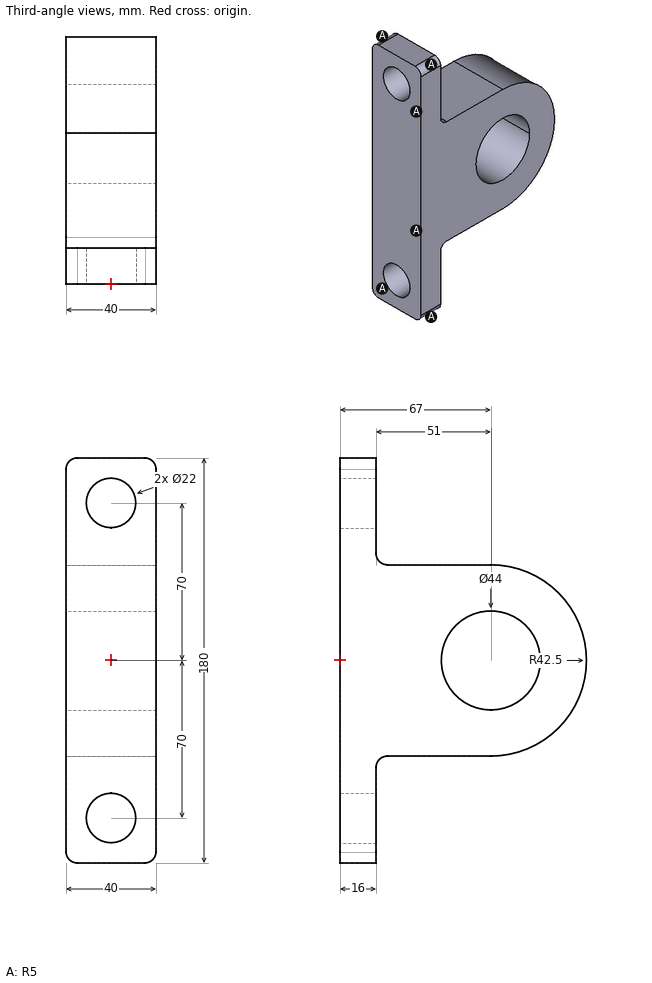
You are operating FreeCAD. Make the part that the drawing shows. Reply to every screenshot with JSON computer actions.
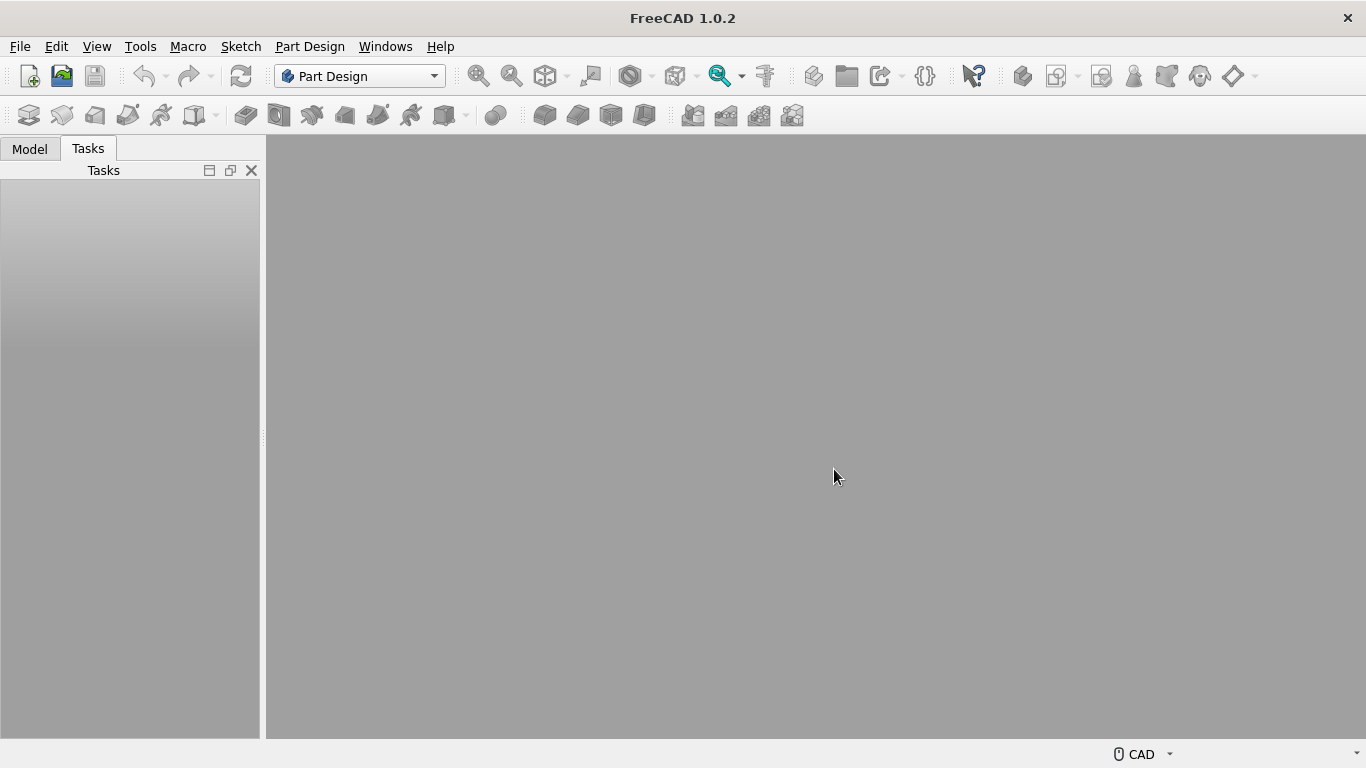
{"action": "left_click", "coordinate": [29, 76]}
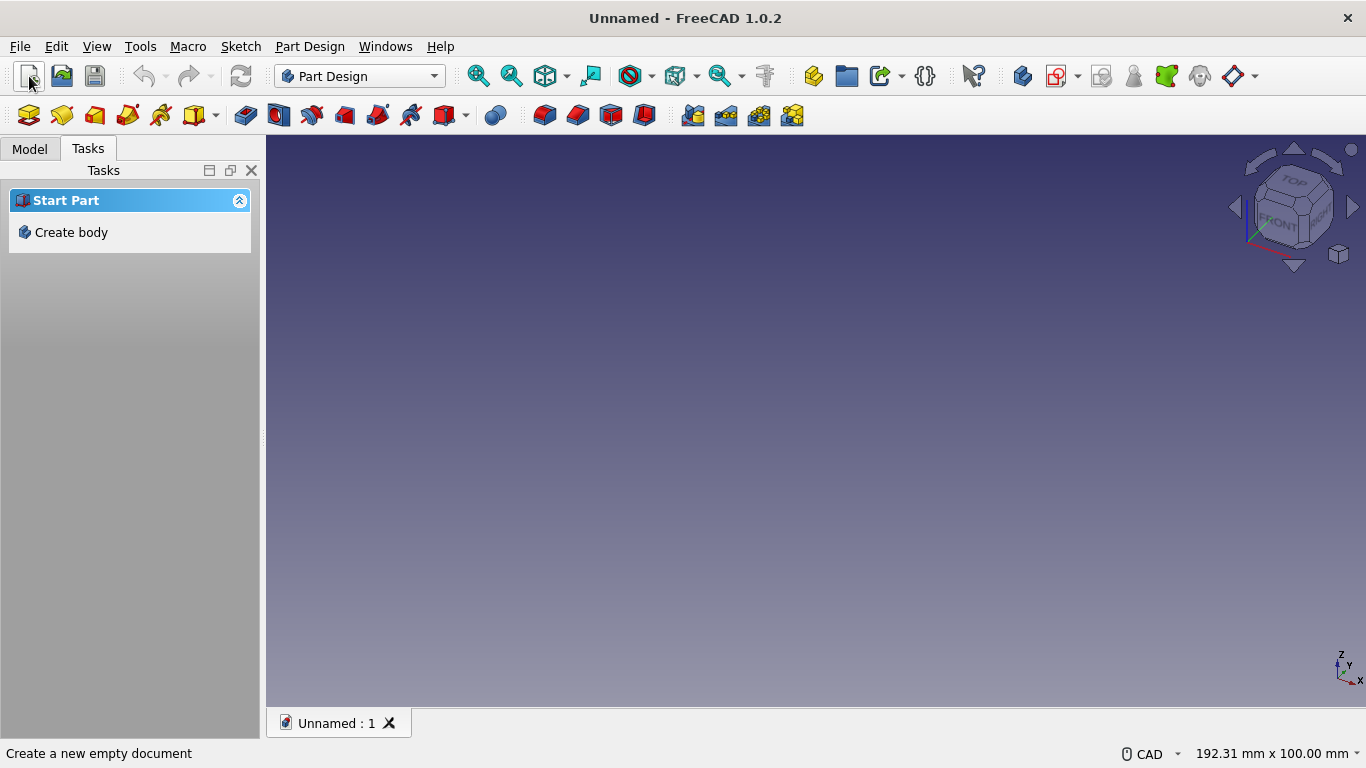
{"action": "left_click", "coordinate": [1056, 76]}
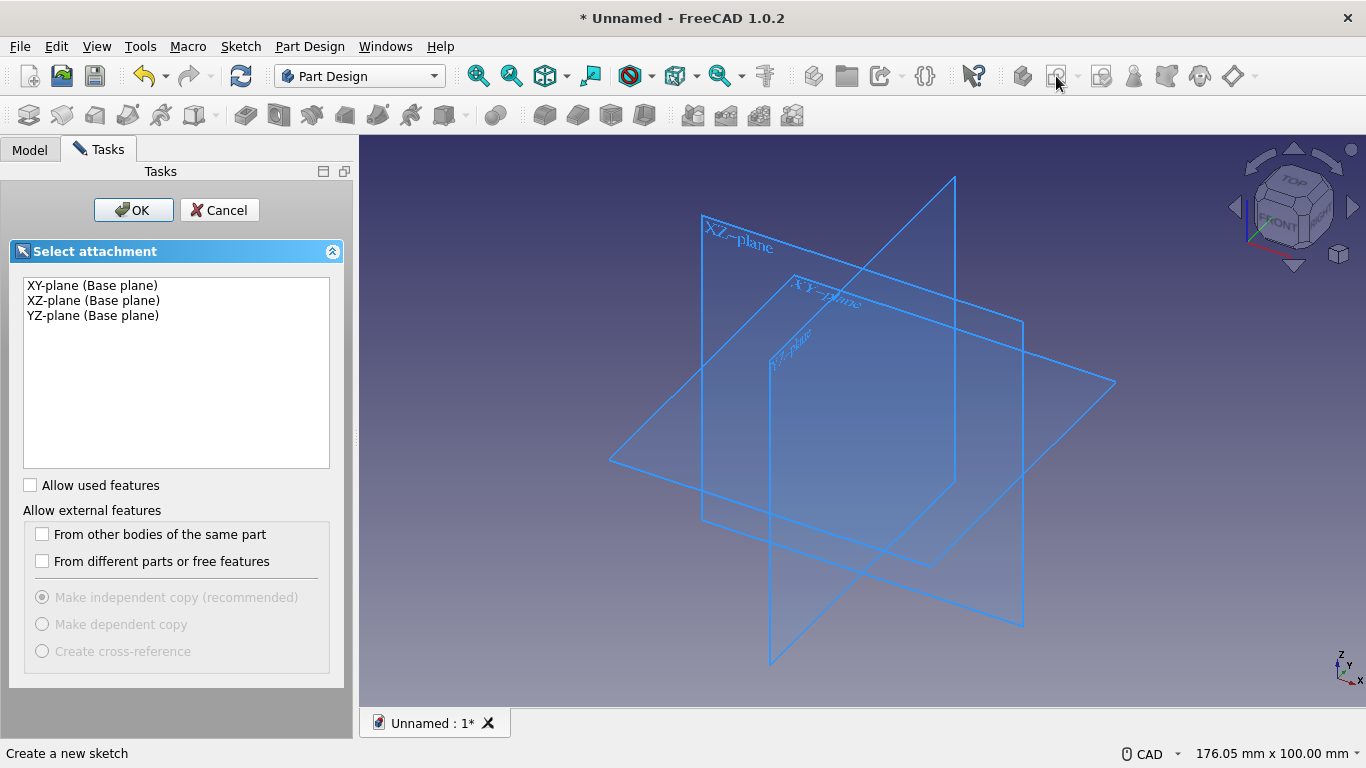
{"action": "left_click", "coordinate": [84, 300]}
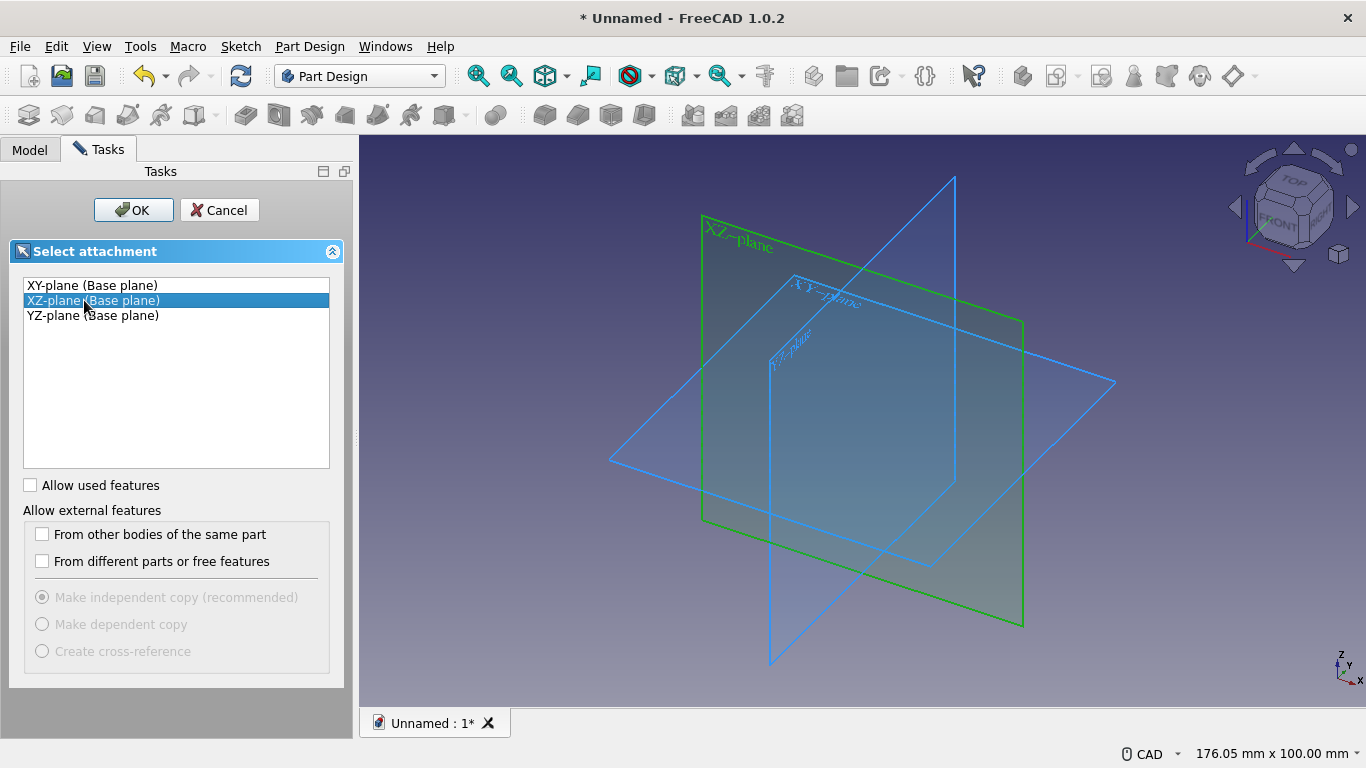
{"action": "left_click", "coordinate": [134, 210]}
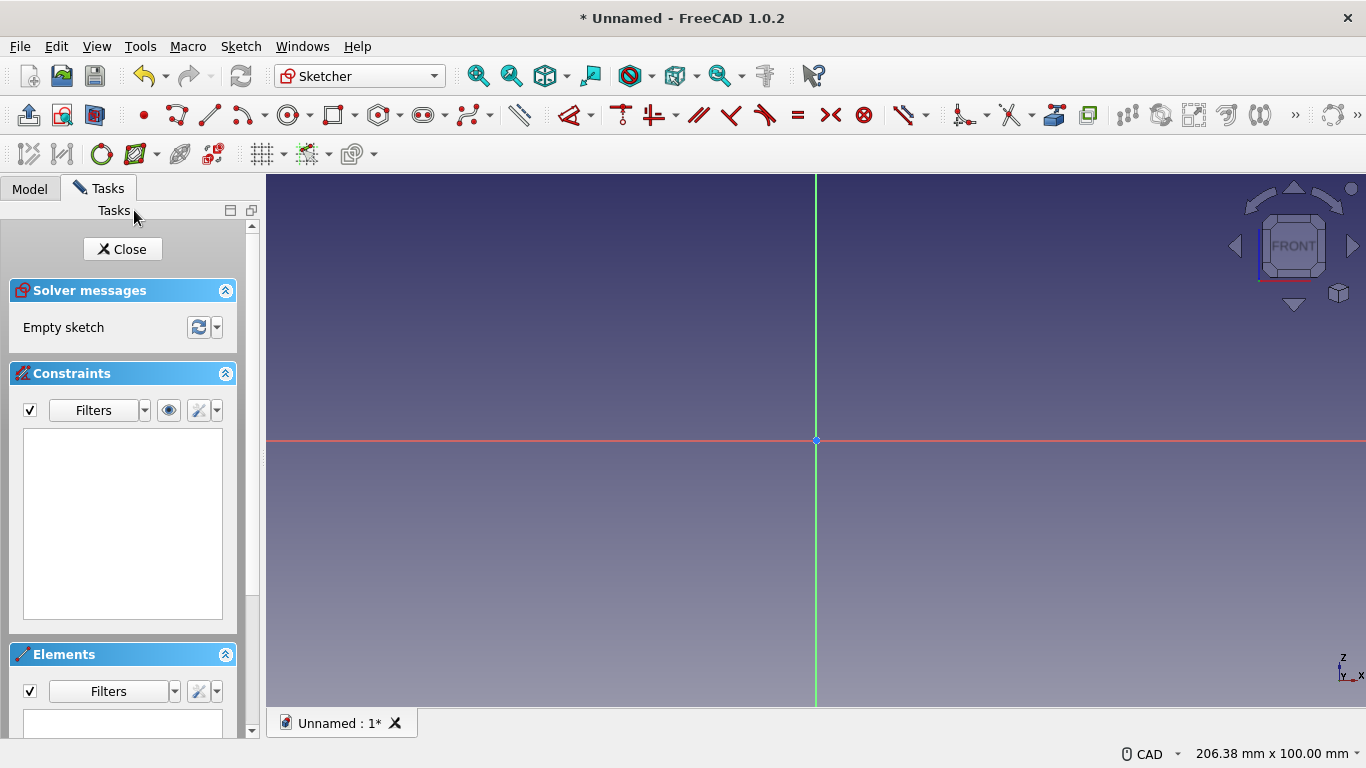
{"action": "scroll", "coordinate": [708, 440], "scroll_direction": "down", "scroll_amount": 5}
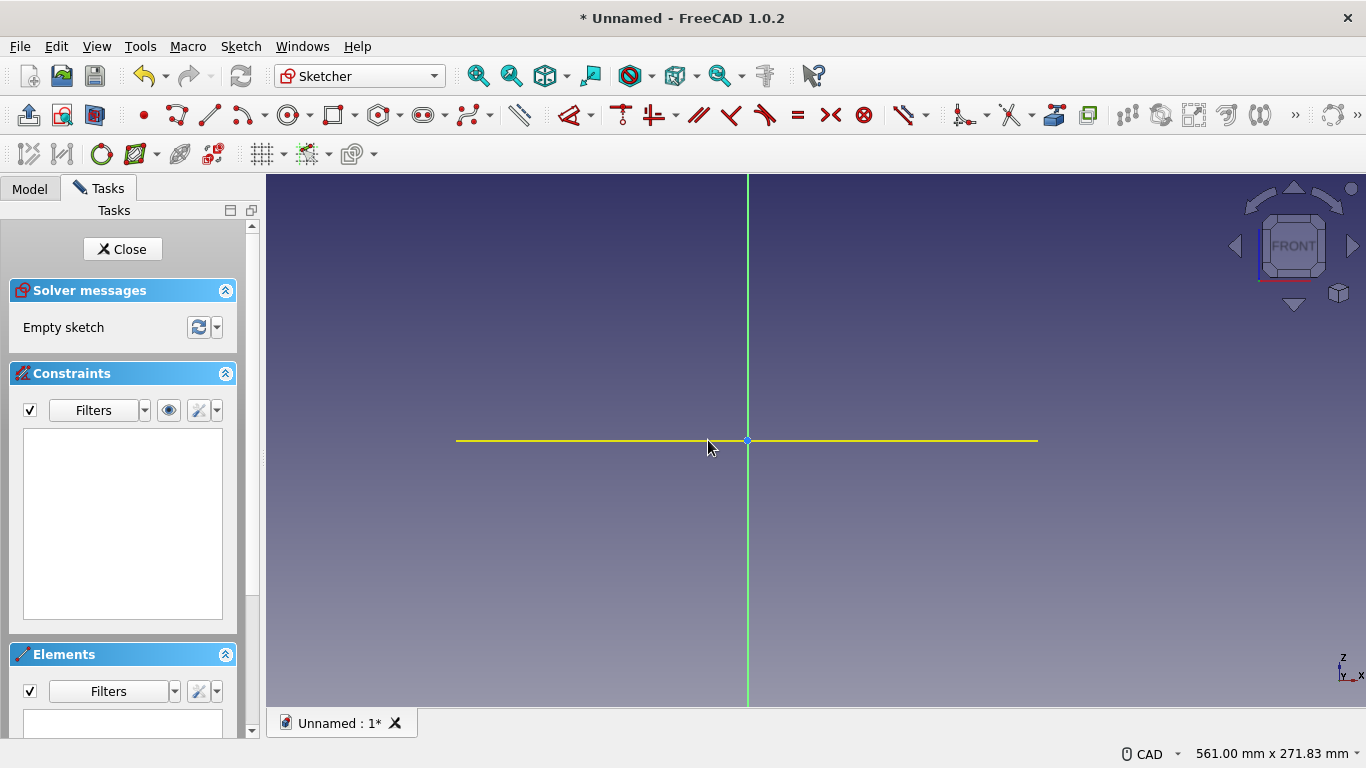
{"action": "left_click", "coordinate": [354, 116]}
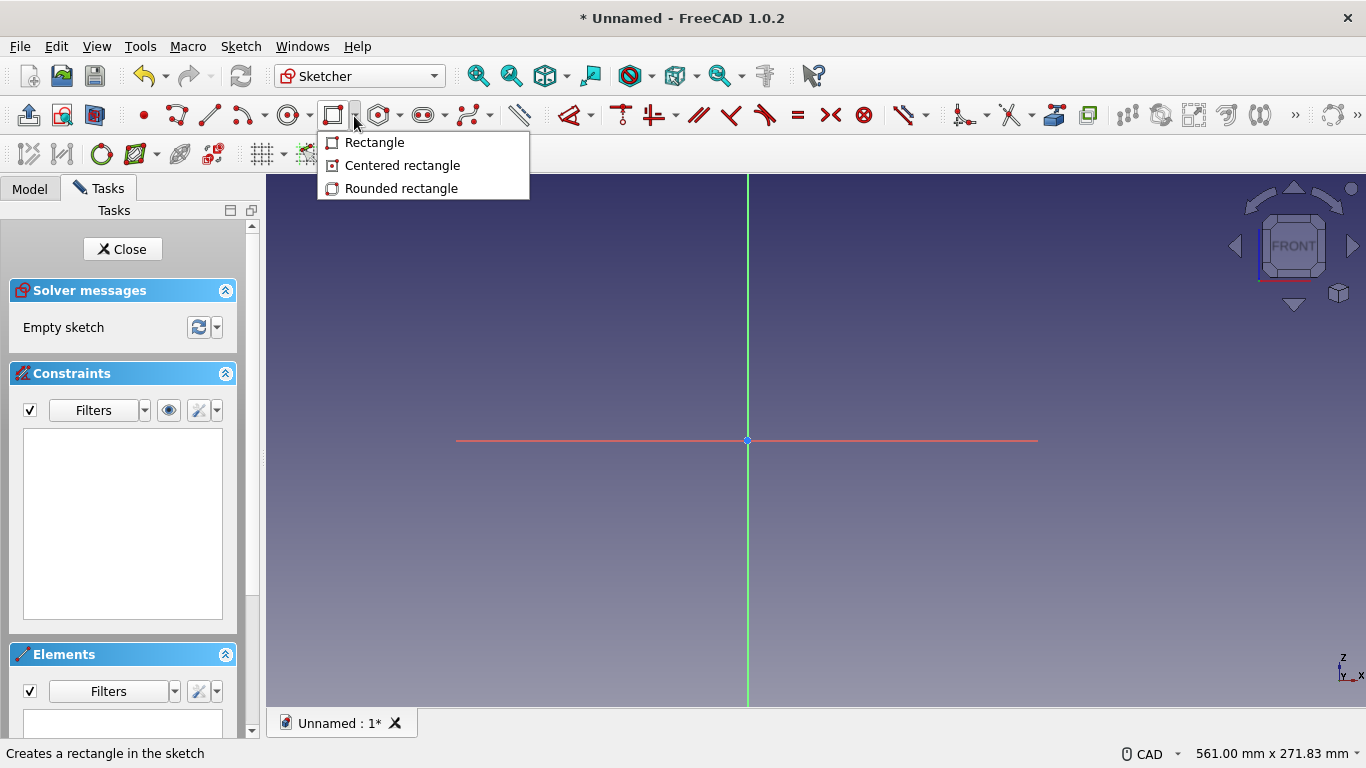
{"action": "left_click", "coordinate": [424, 166]}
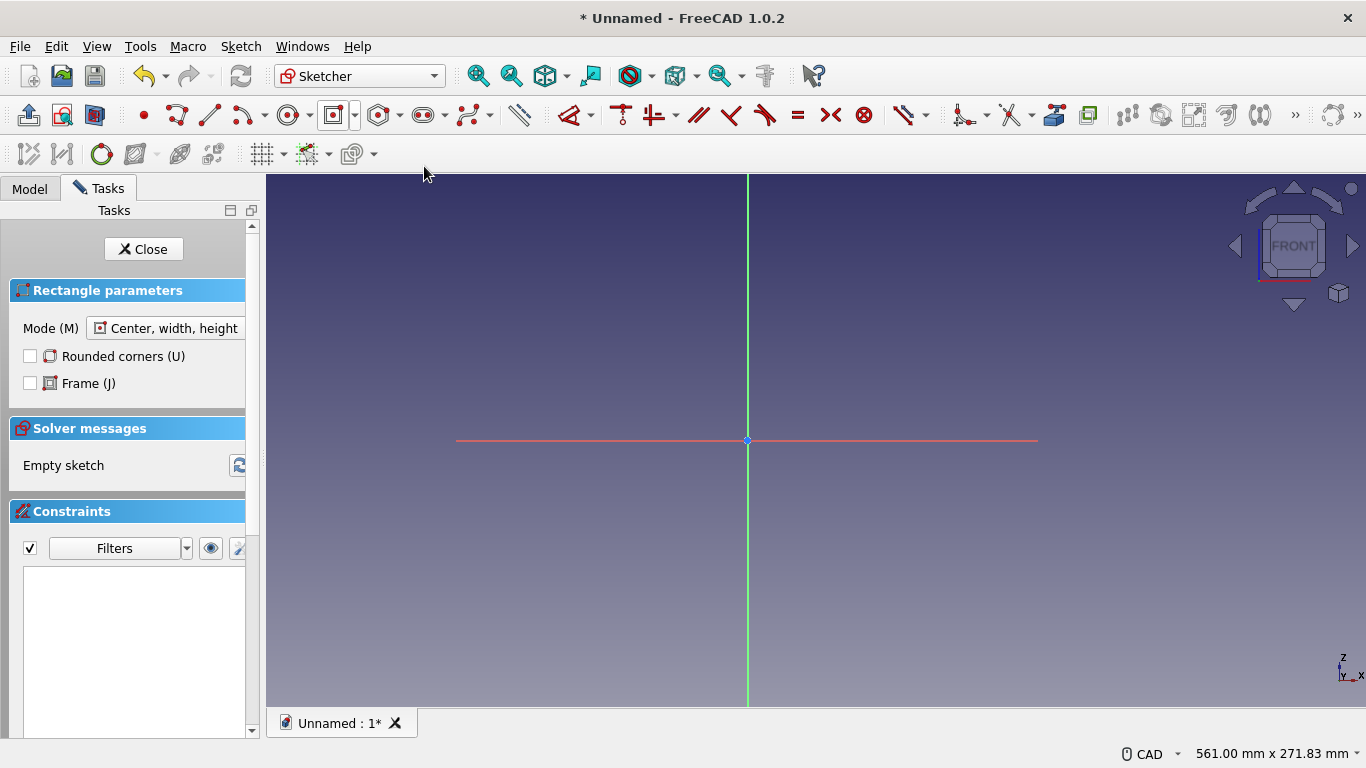
{"action": "left_click", "coordinate": [748, 440]}
{"action": "mouse_move", "coordinate": [787, 264]}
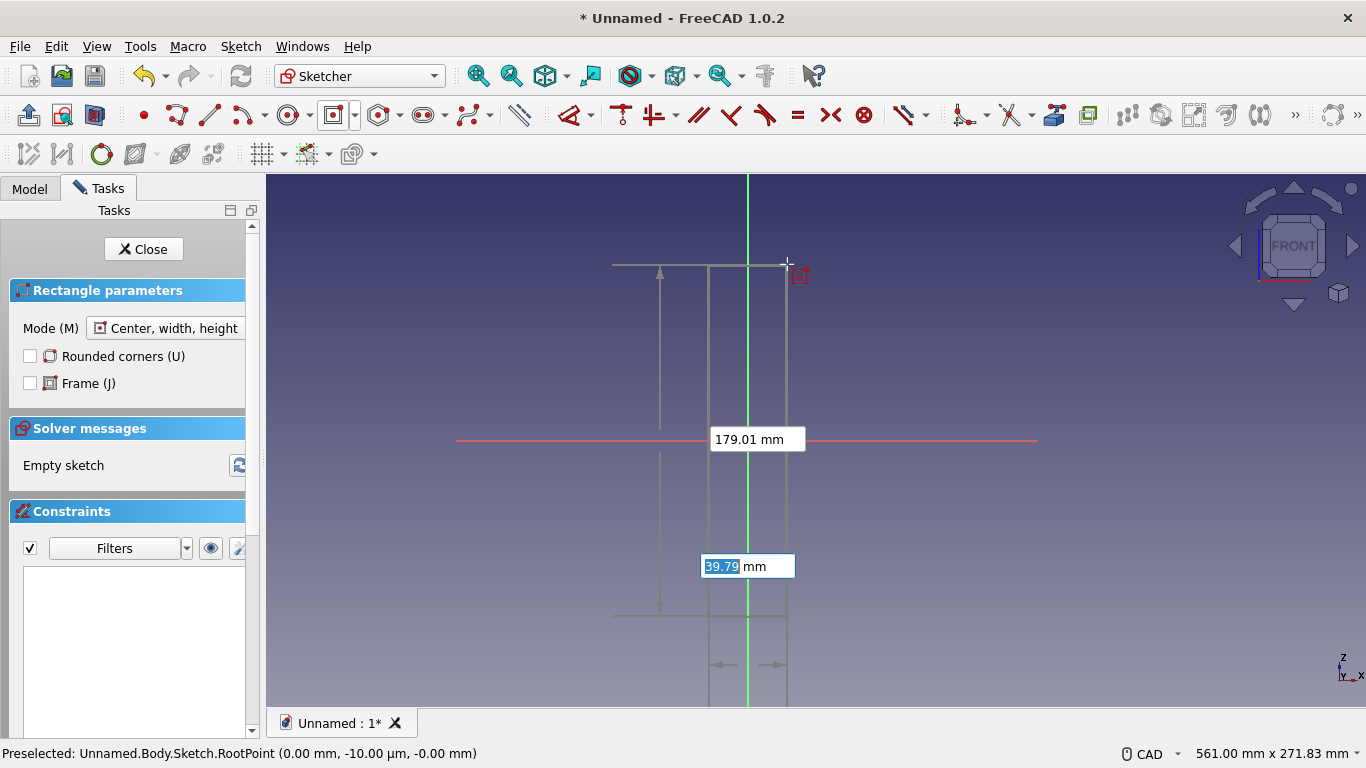
{"action": "type", "text": "40"}
{"action": "key", "text": "Tab"}
{"action": "type", "text": "180"}
{"action": "key", "text": "Return"}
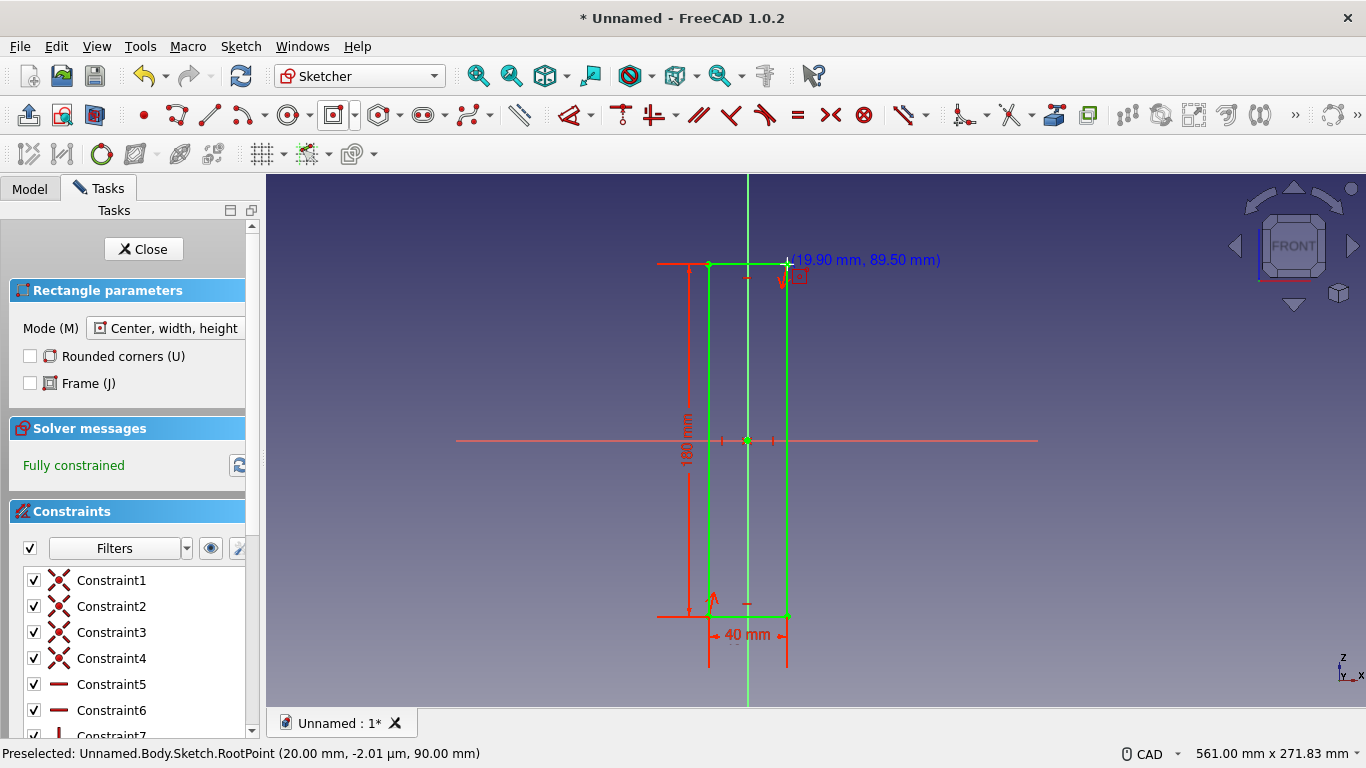
{"action": "key", "text": "g c"}